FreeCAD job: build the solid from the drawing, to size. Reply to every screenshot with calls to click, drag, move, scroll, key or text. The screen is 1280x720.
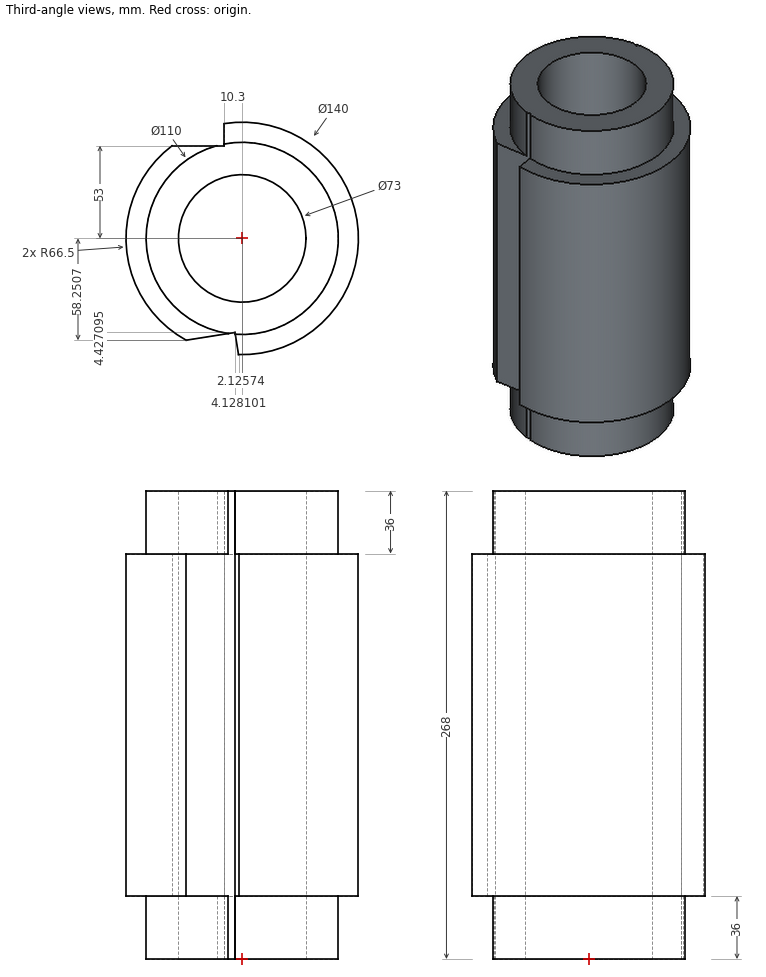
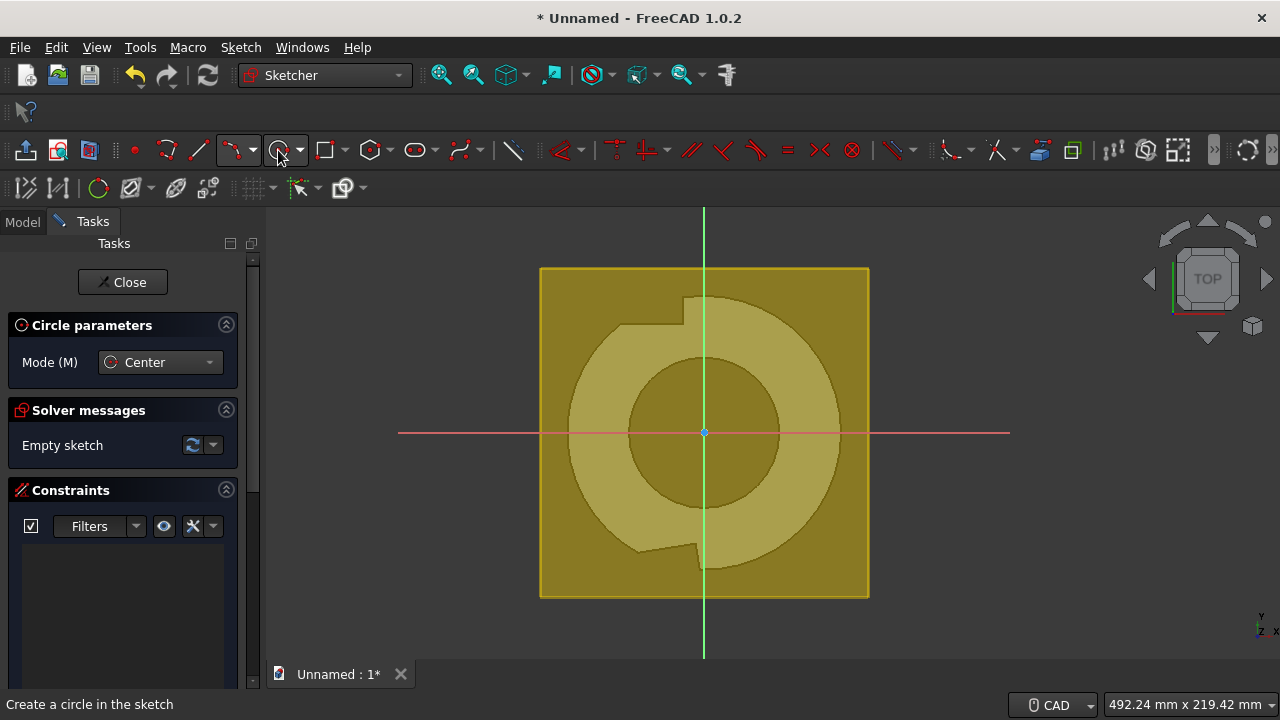
click(704, 433)
click(806, 331)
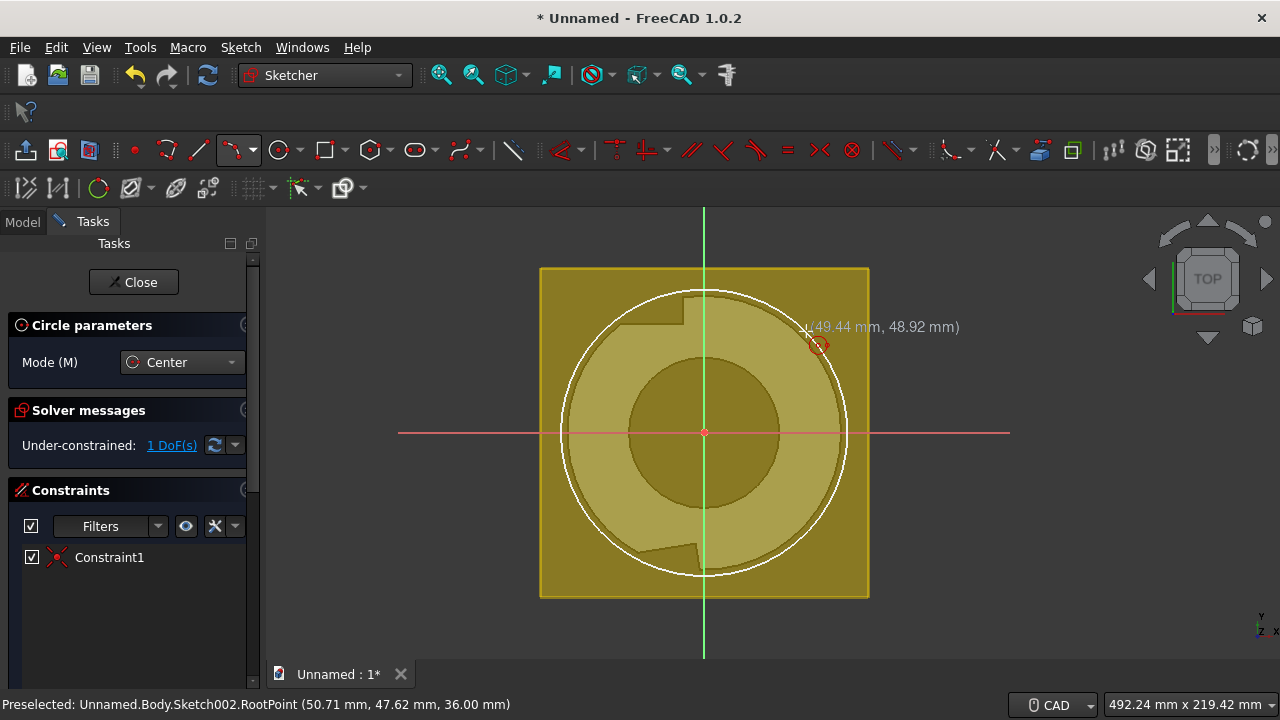
click(704, 433)
click(784, 353)
key(Escape)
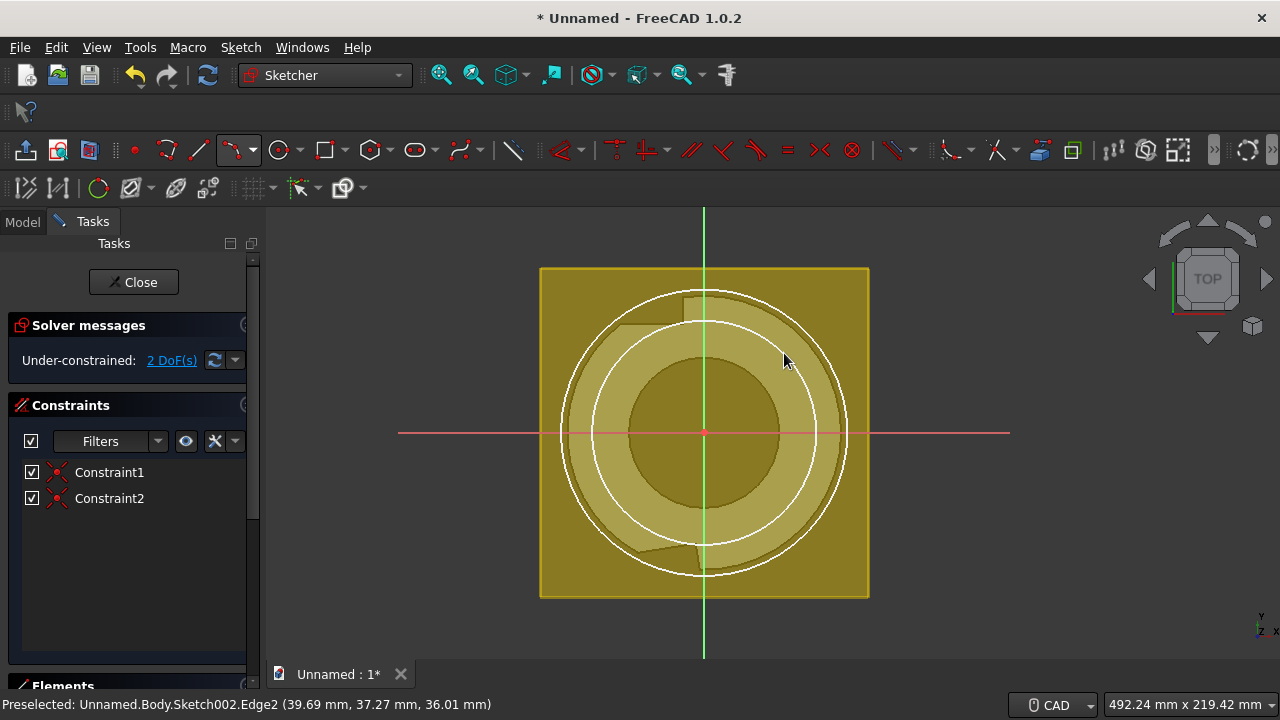
click(560, 150)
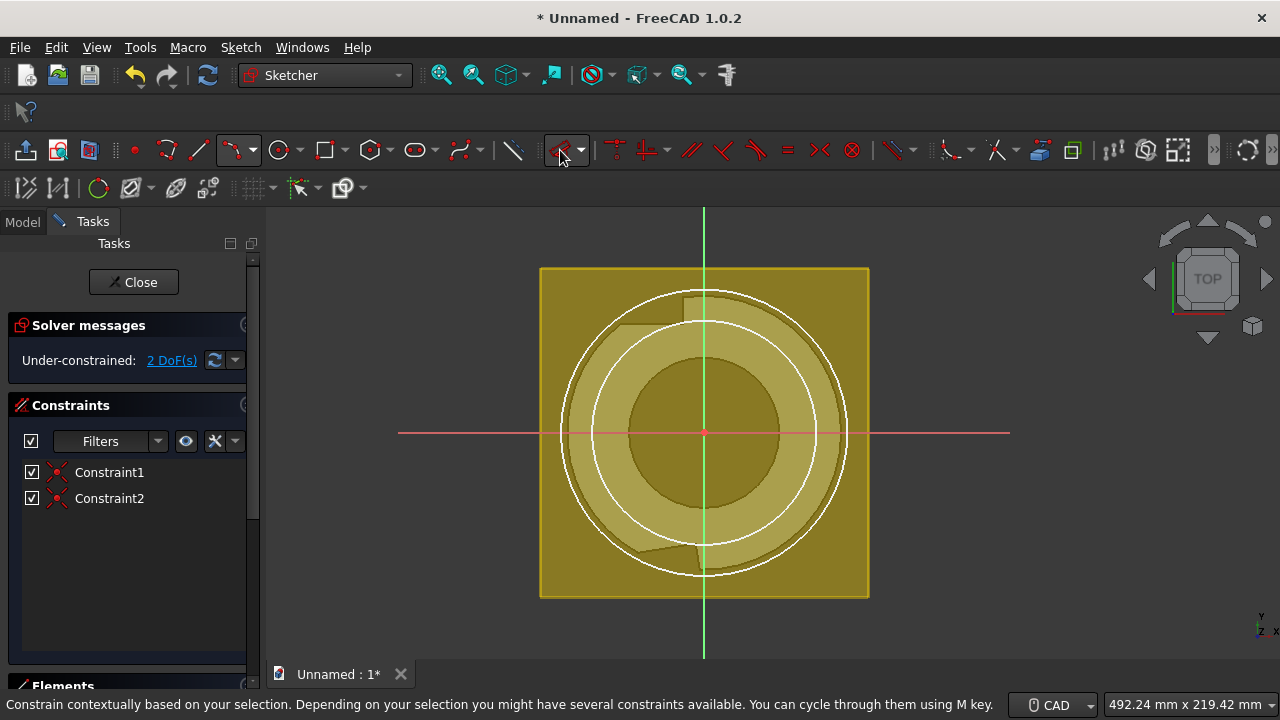
click(805, 331)
click(828, 308)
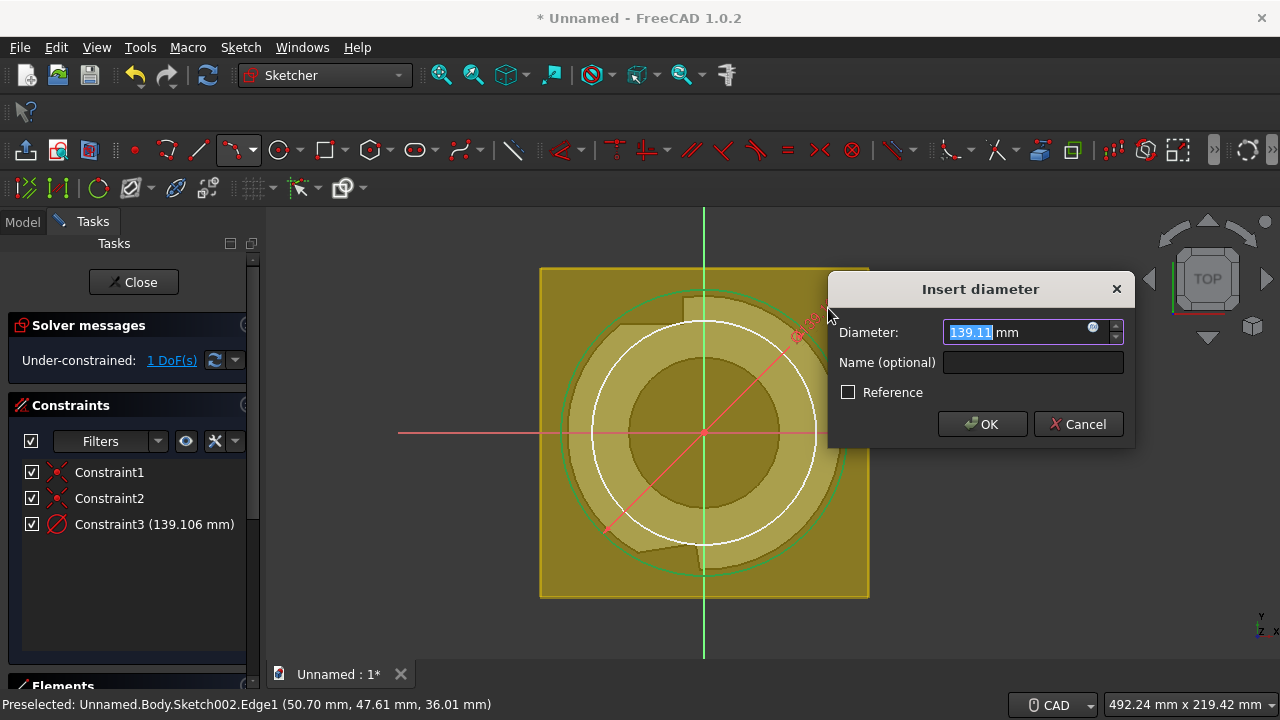
text(140)
key(Return)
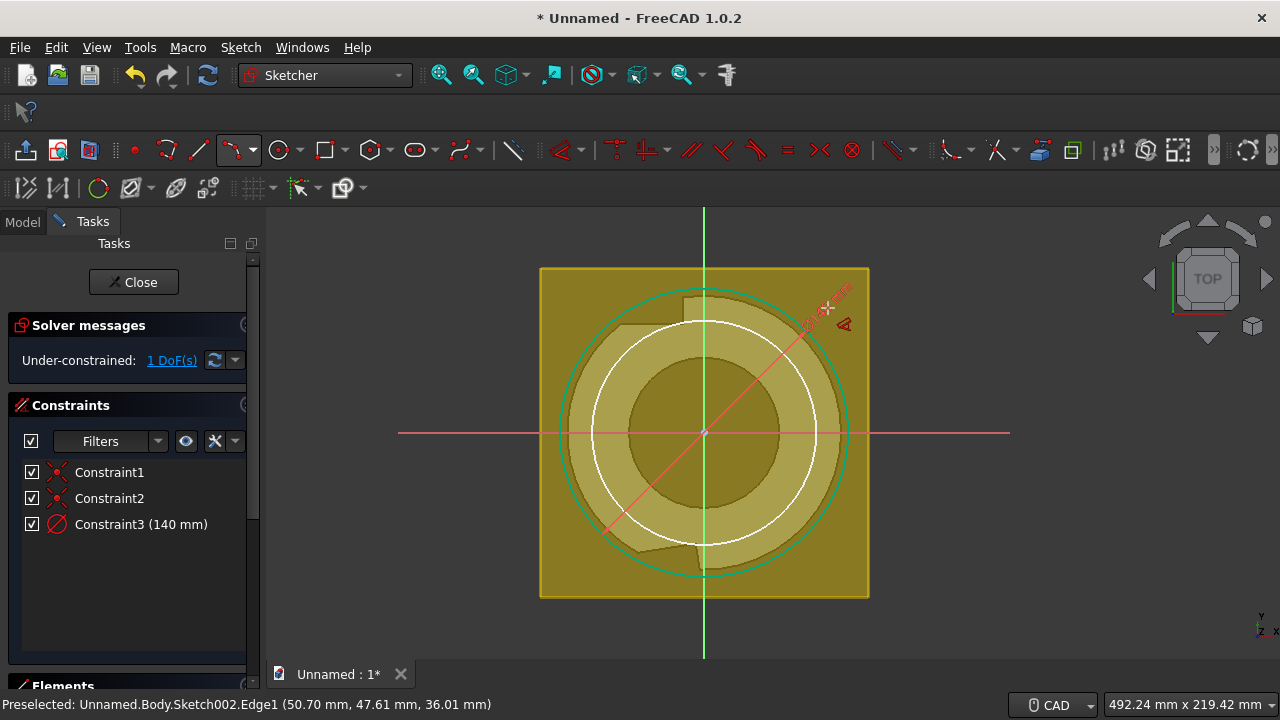
click(783, 353)
click(864, 385)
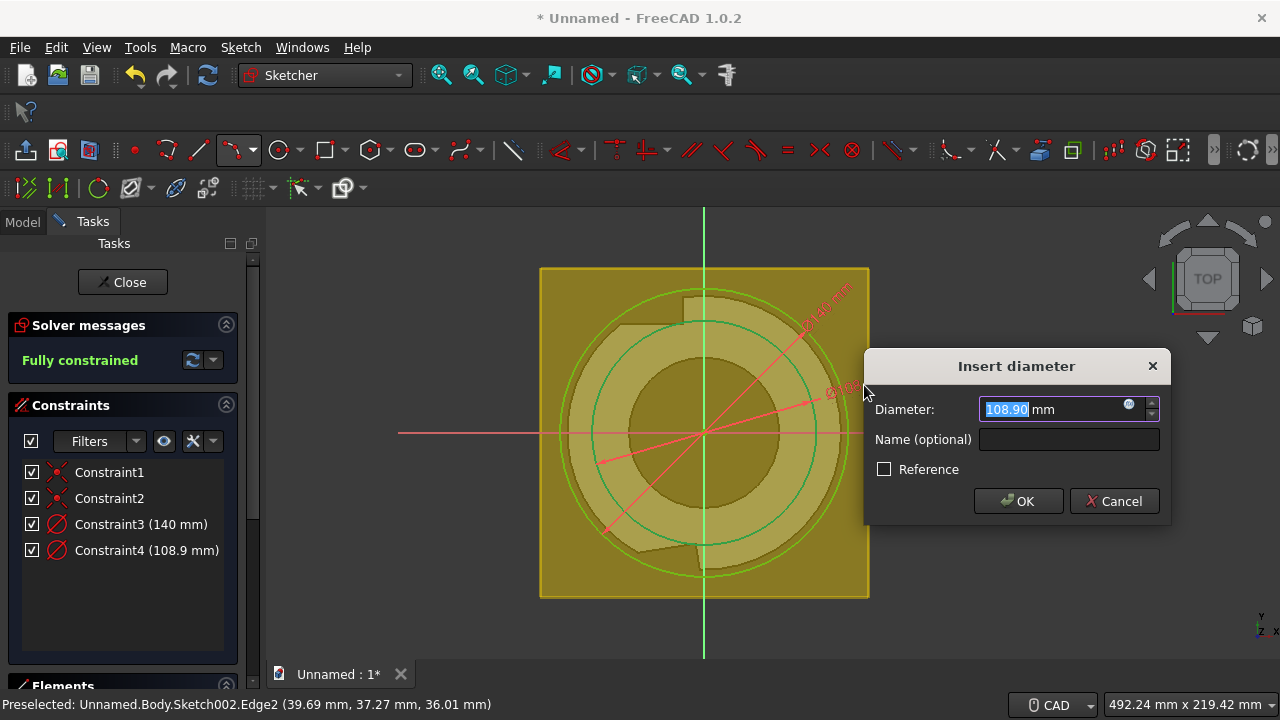
text(110)
key(Return)
key(Escape)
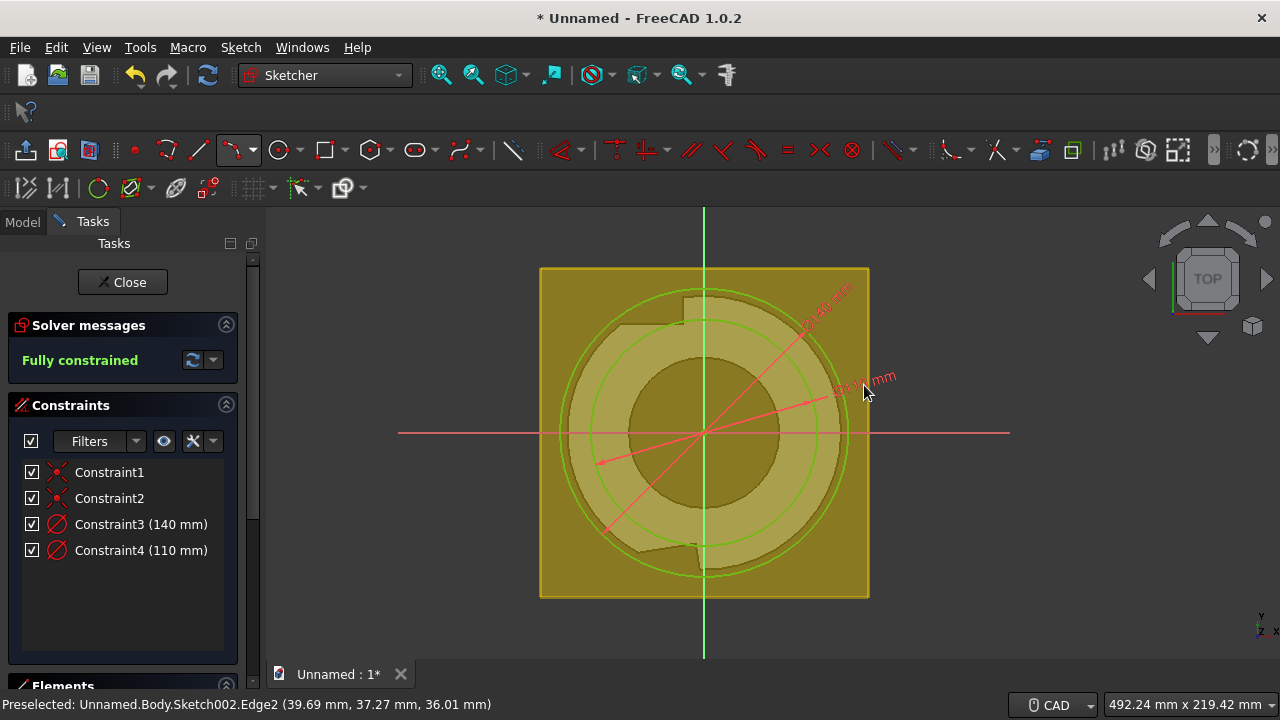
click(123, 282)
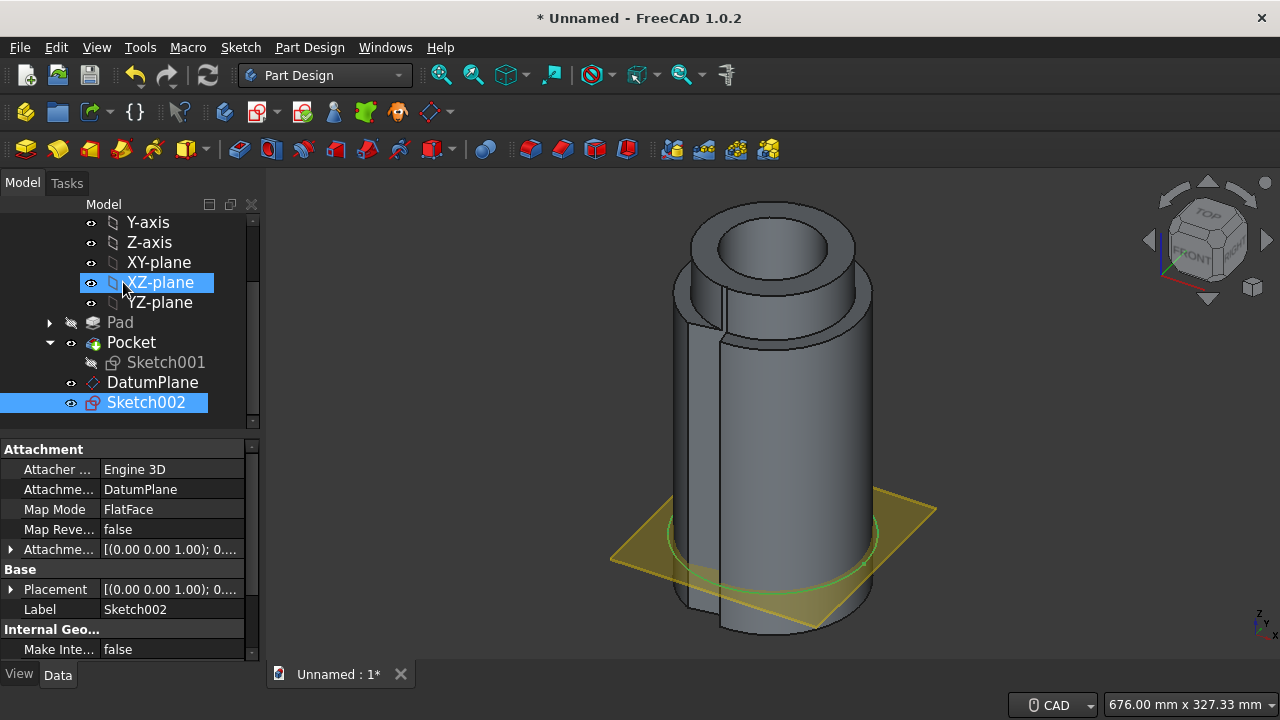
click(240, 150)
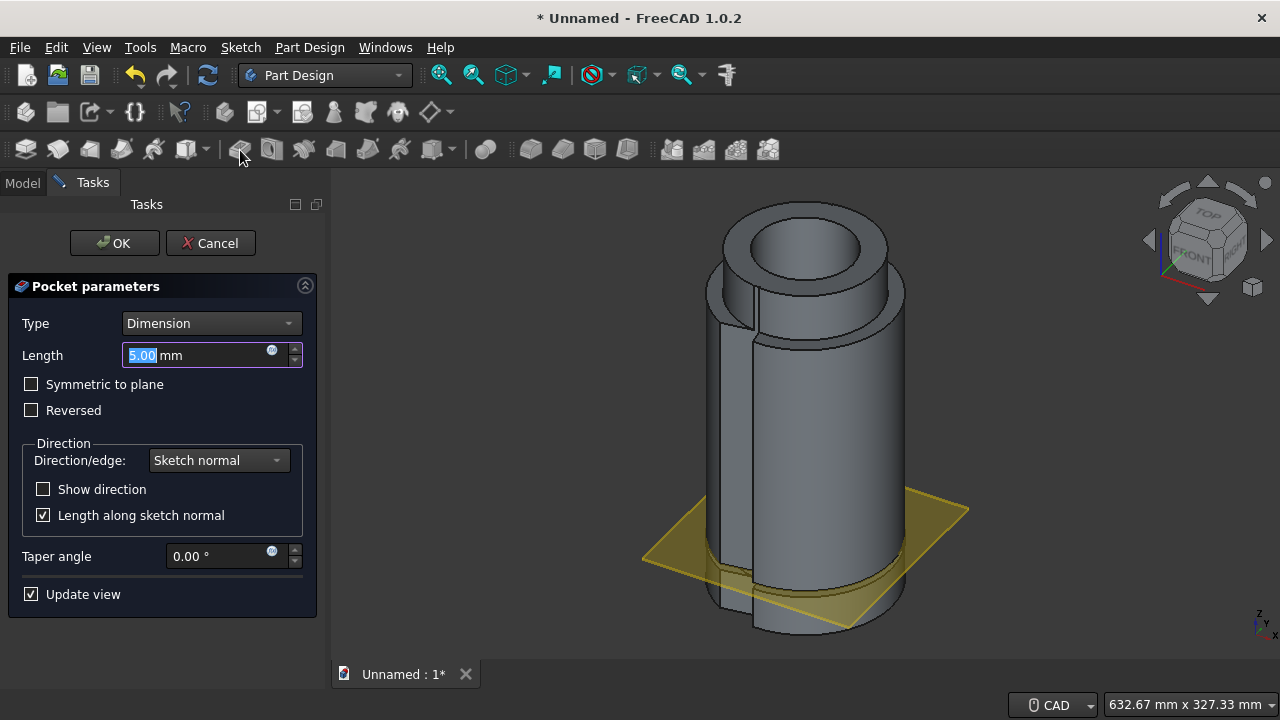
text(36)
key(Tab)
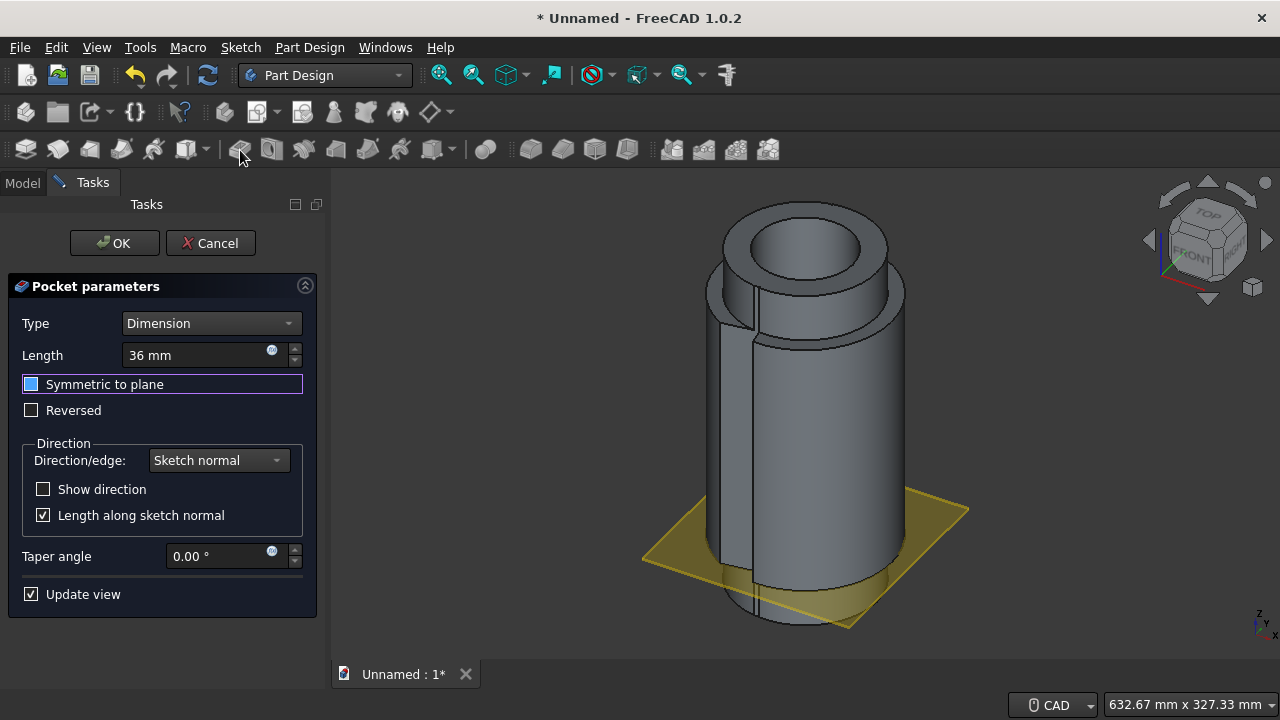
click(115, 243)